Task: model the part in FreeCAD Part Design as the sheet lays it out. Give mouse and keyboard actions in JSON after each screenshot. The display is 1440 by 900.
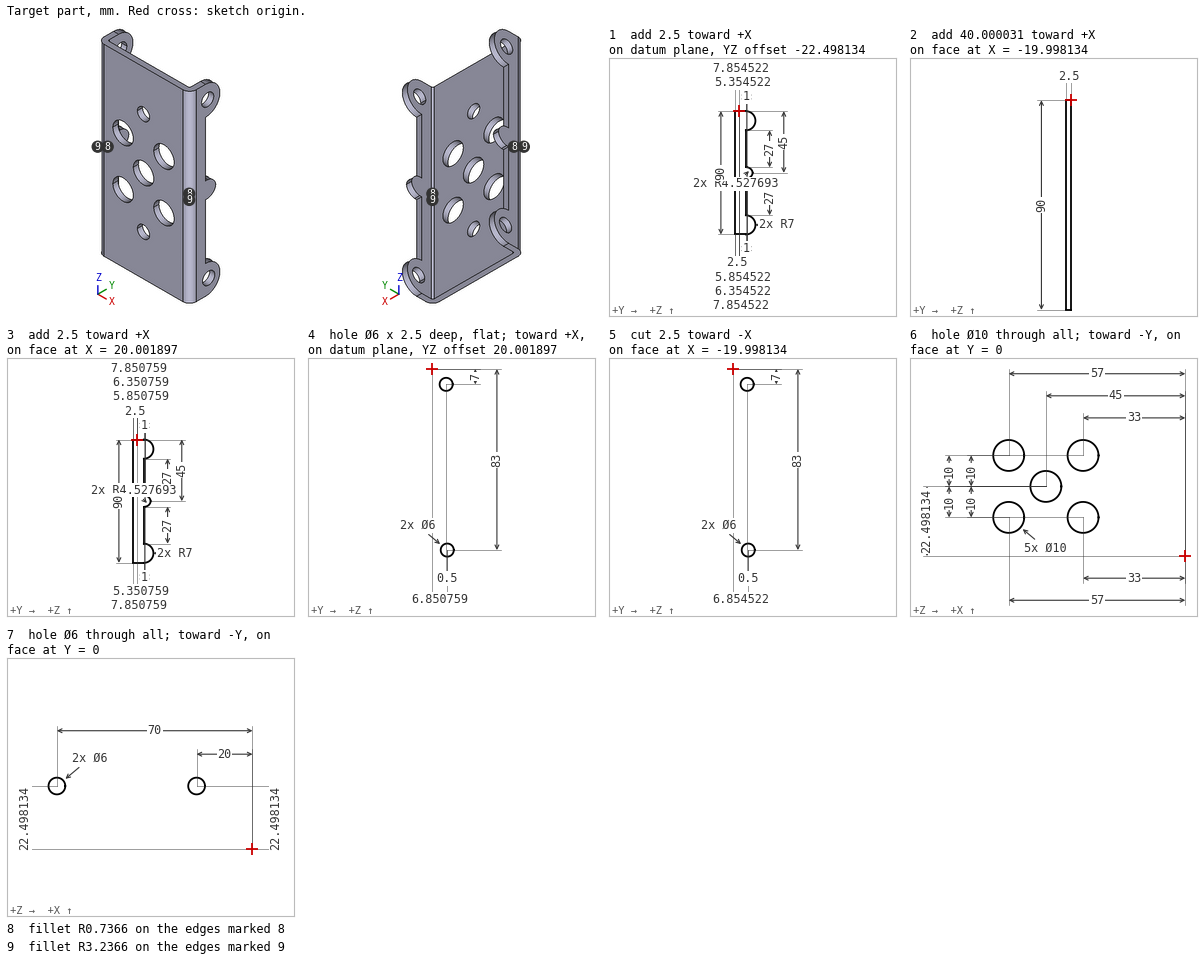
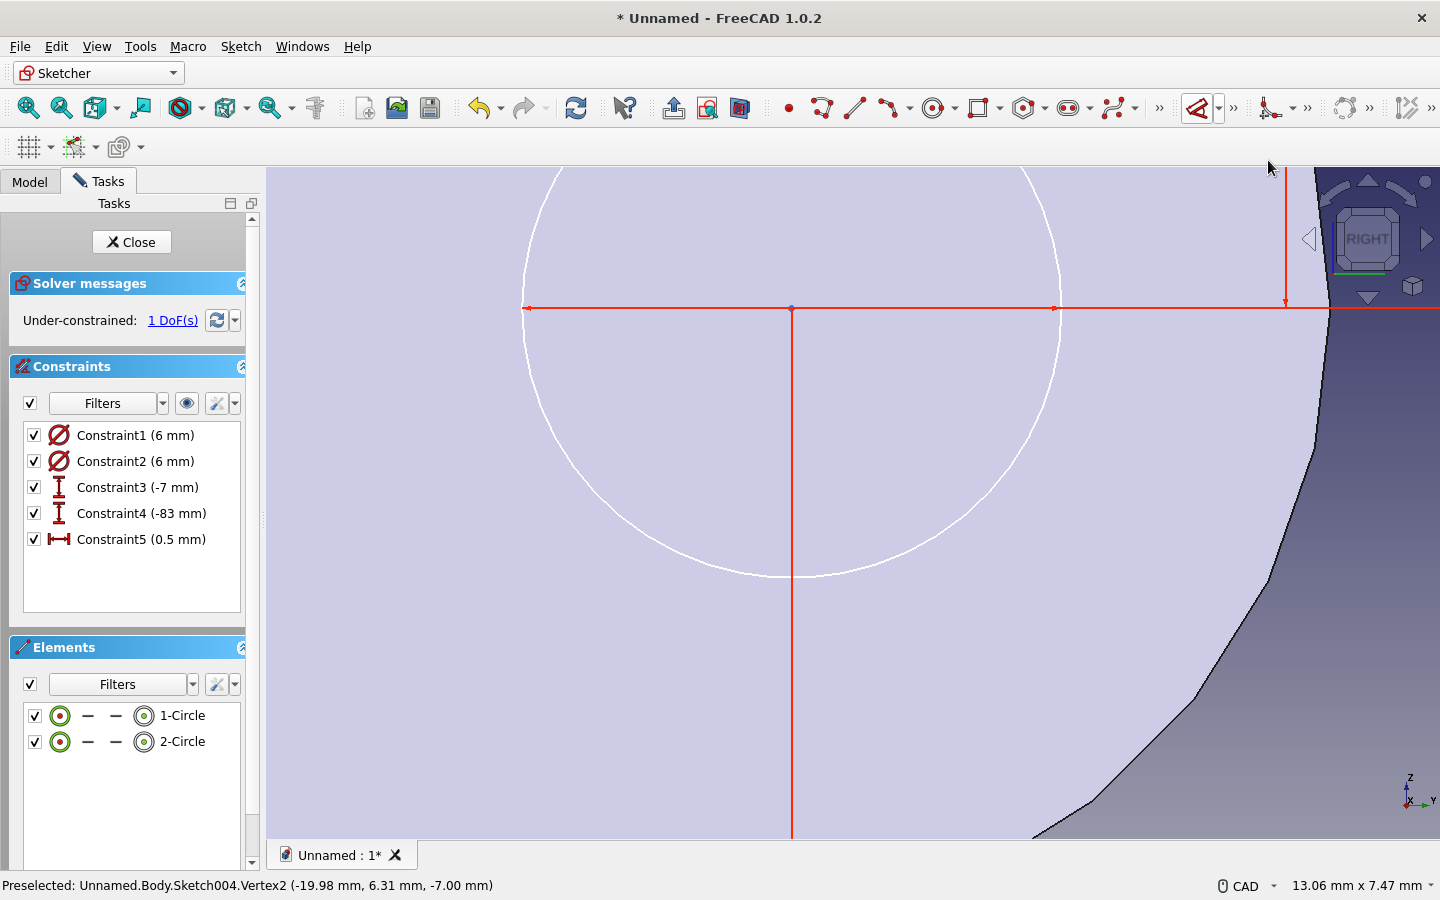
{"action": "scroll", "coordinate": [792, 306], "scroll_direction": "down", "scroll_amount": 14}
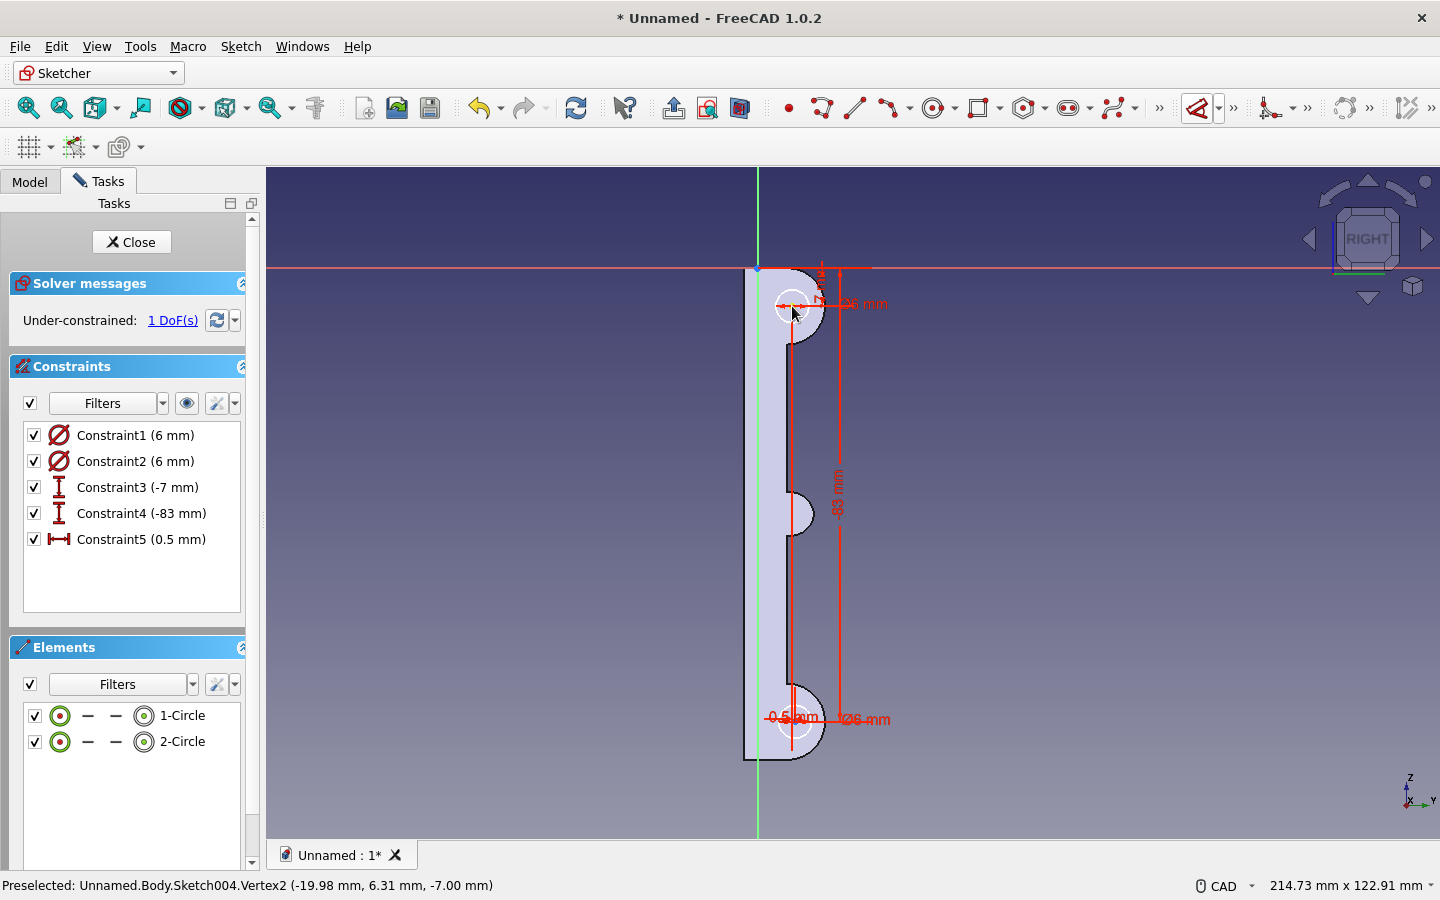
{"action": "left_click", "coordinate": [795, 722]}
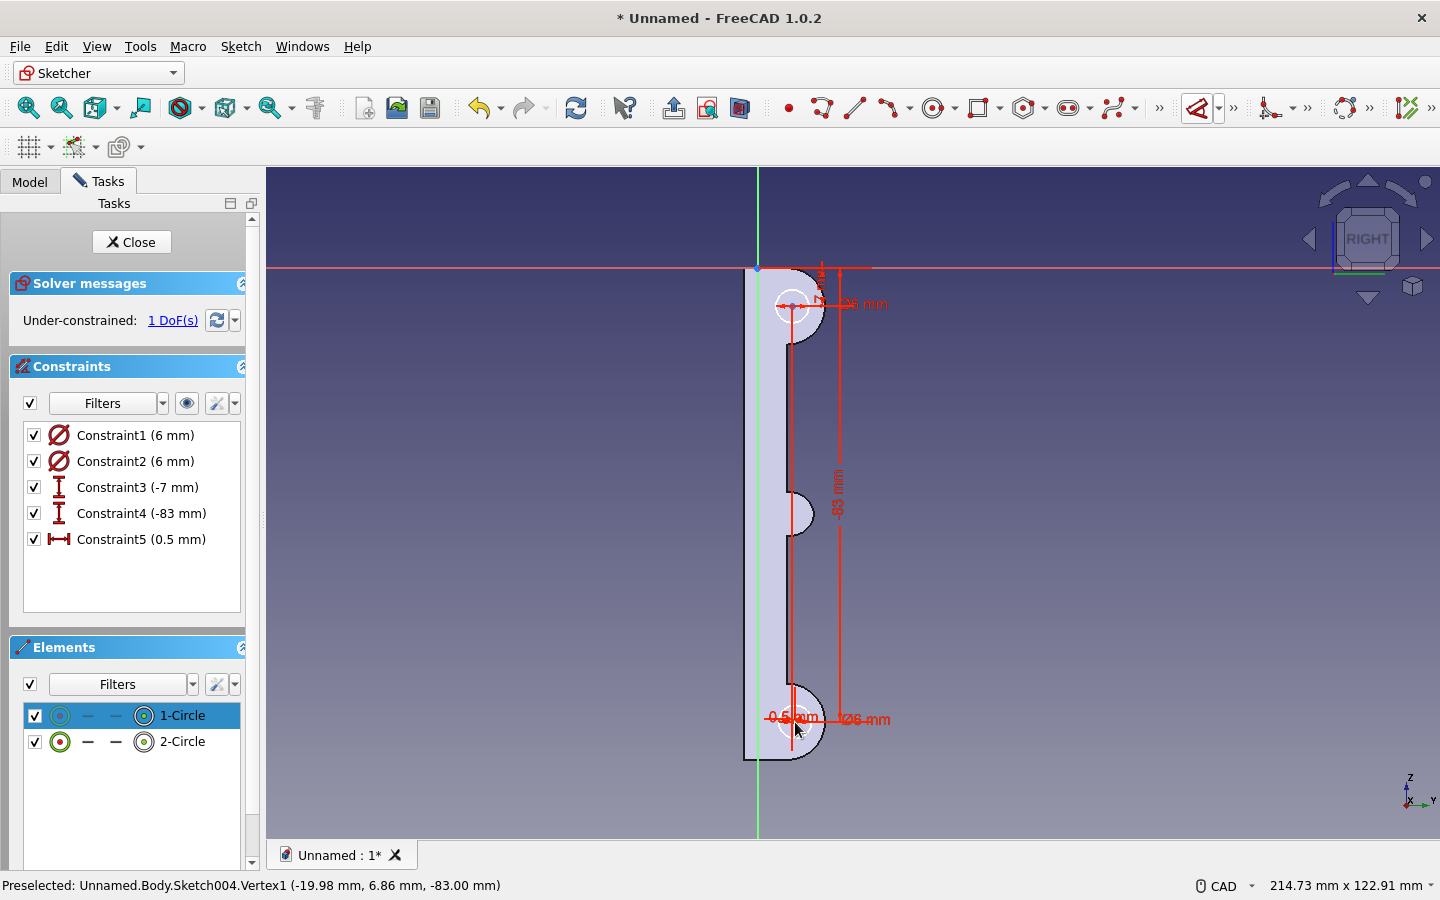
{"action": "left_click", "coordinate": [1218, 108]}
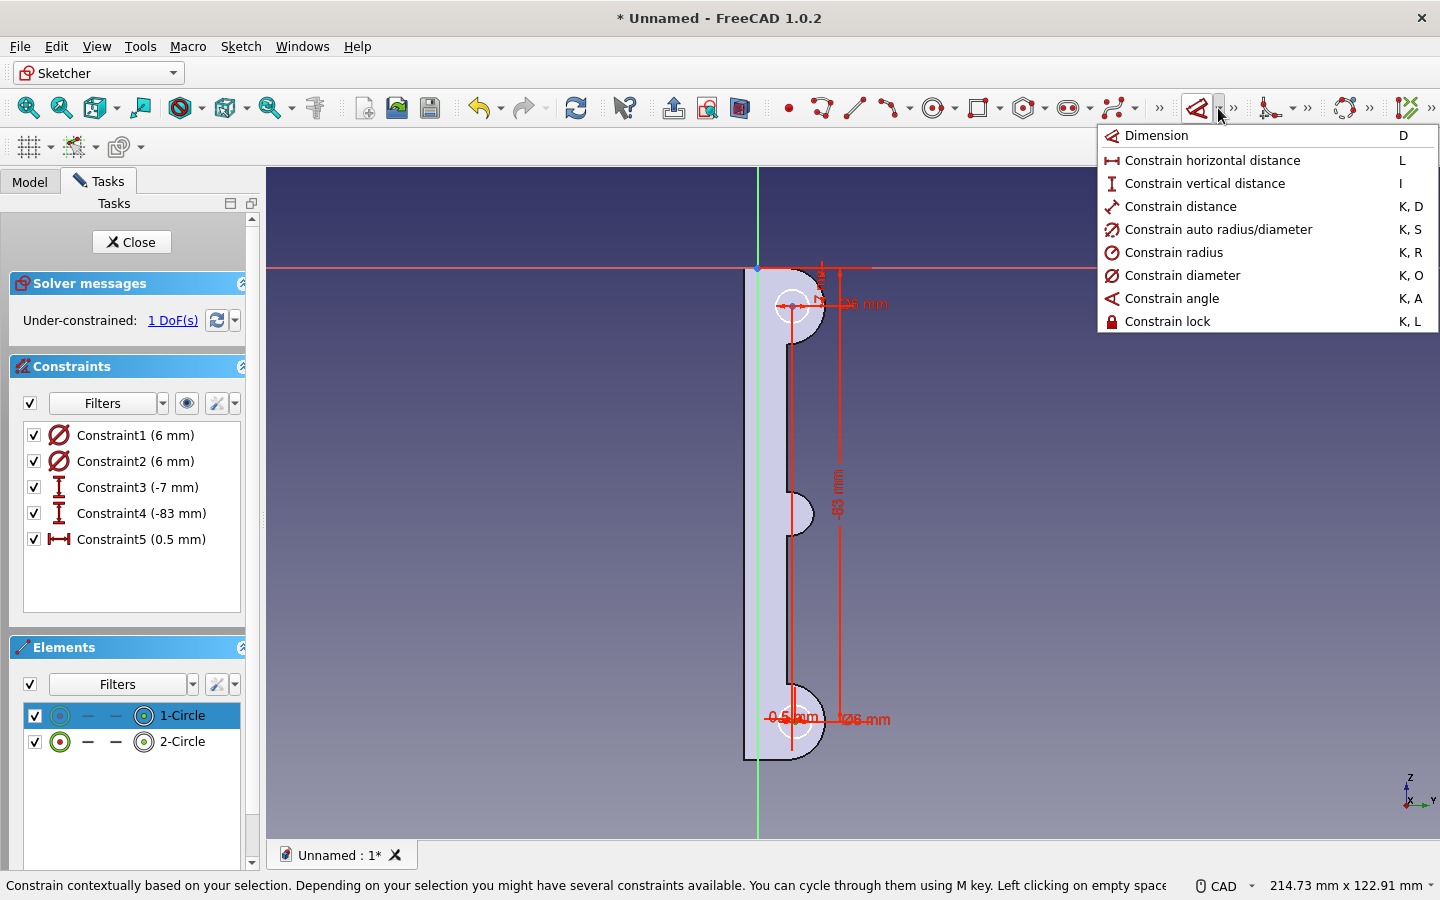
{"action": "left_click", "coordinate": [1268, 160]}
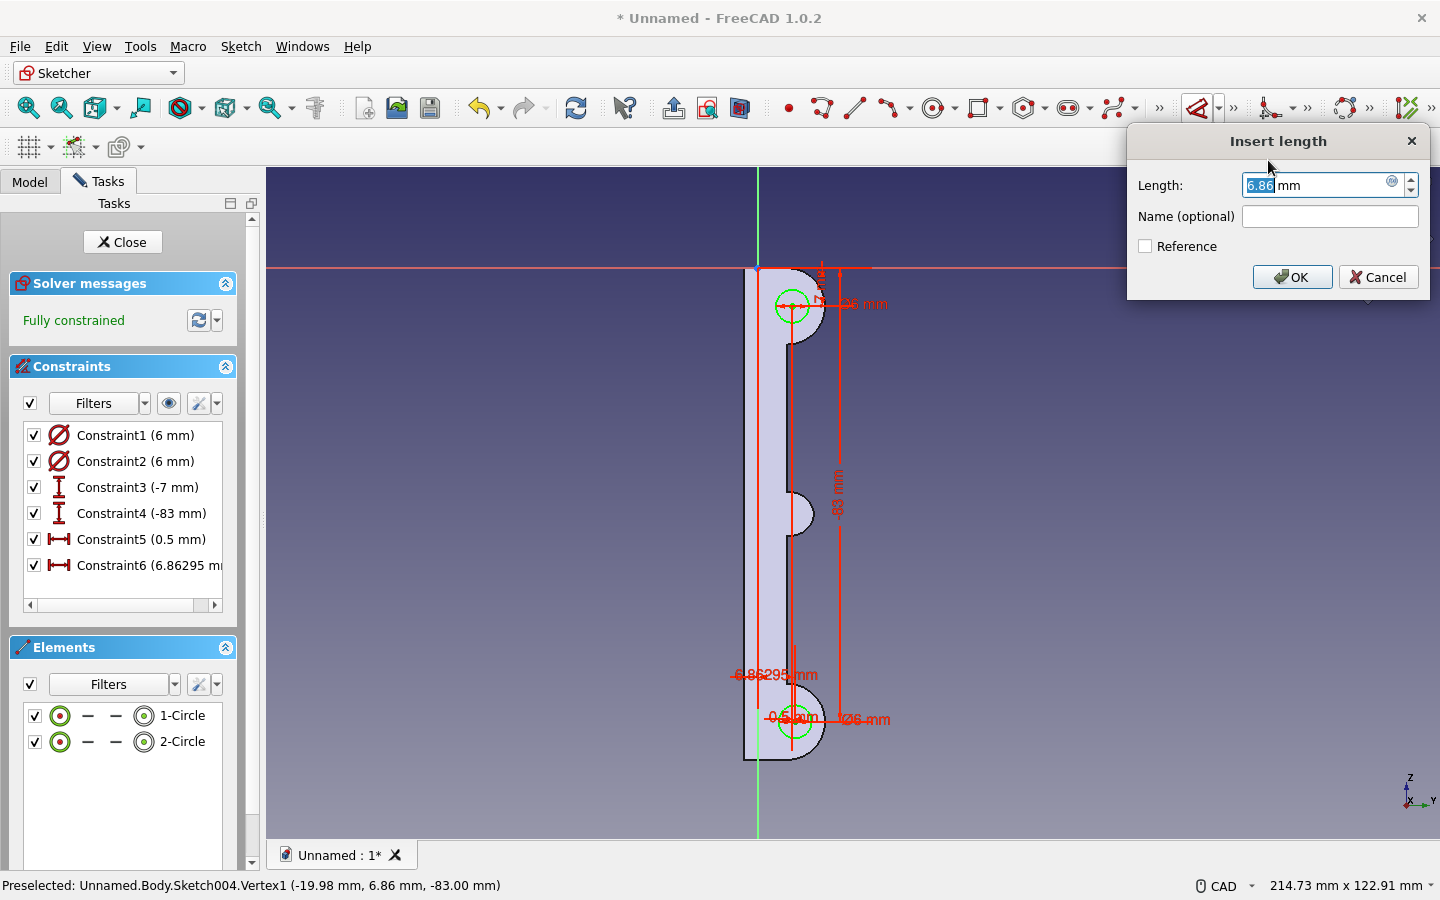
{"action": "type", "text": "6.854522"}
{"action": "key", "text": "Return"}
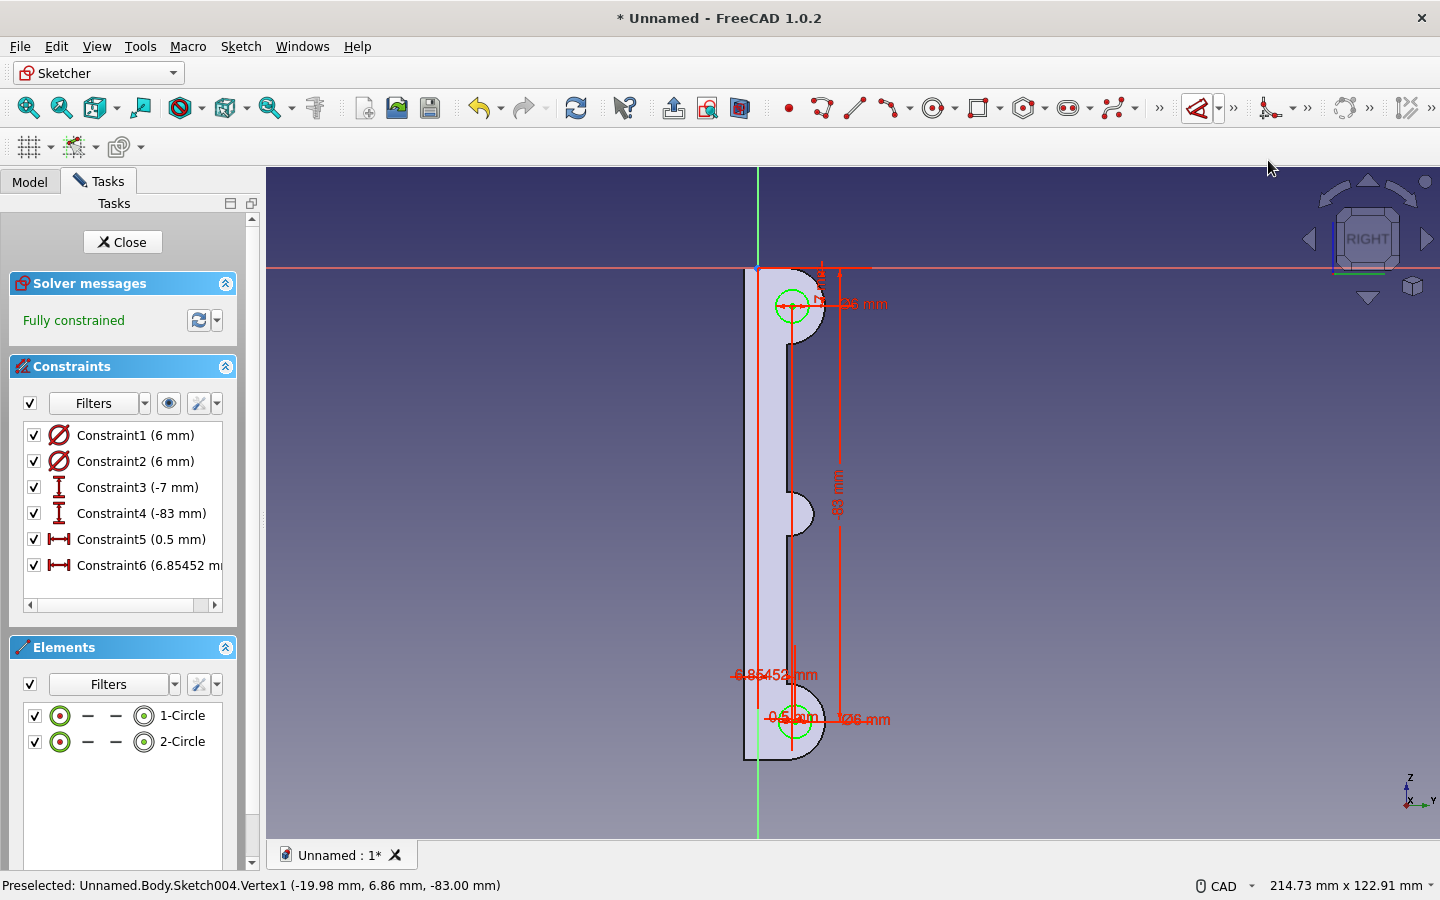
{"action": "left_click", "coordinate": [123, 242]}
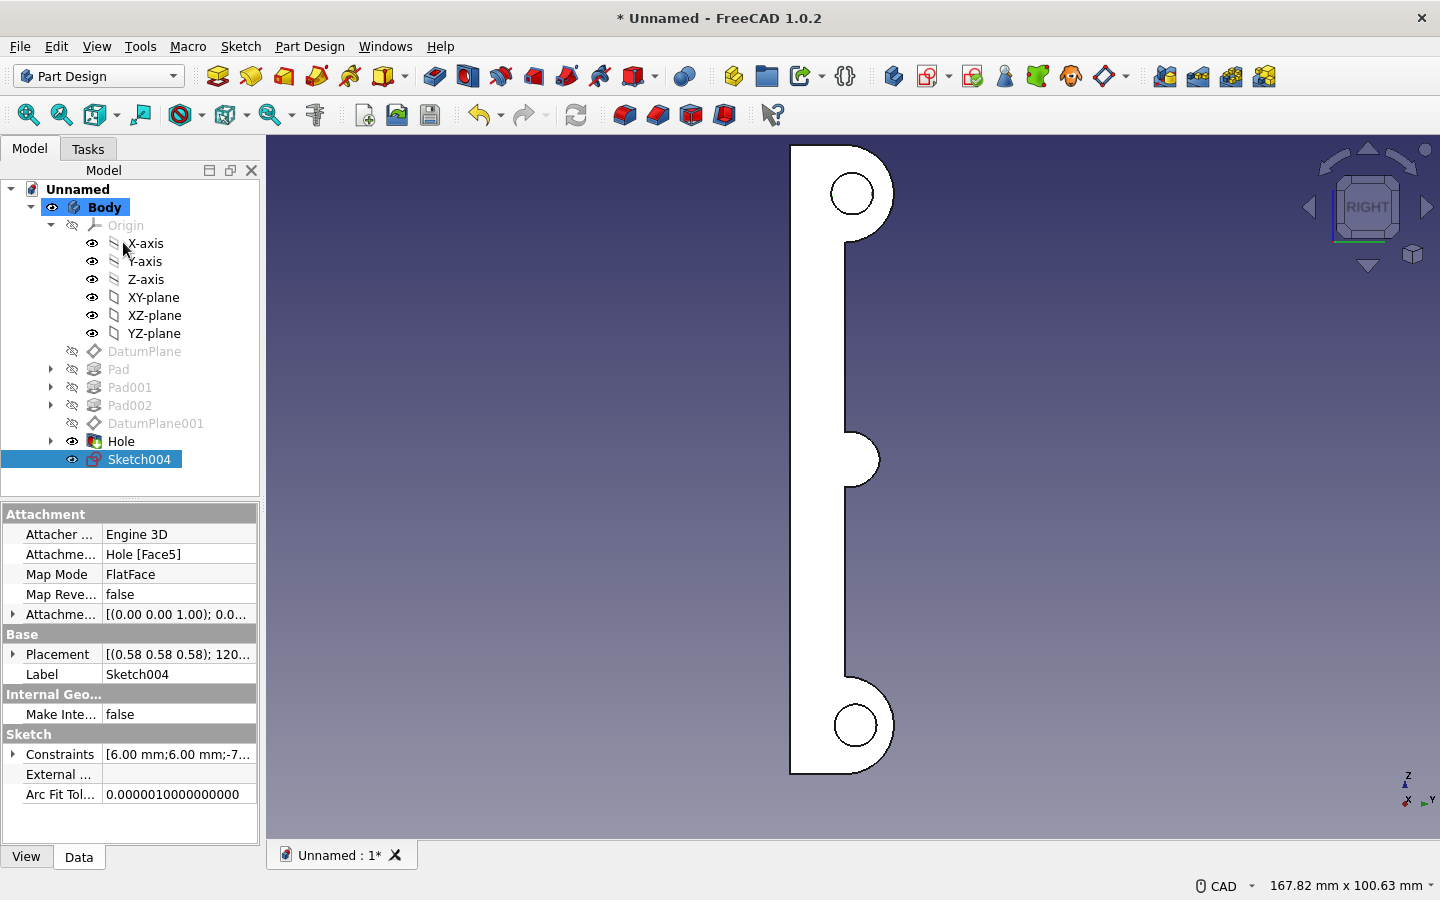
{"action": "left_click", "coordinate": [435, 76]}